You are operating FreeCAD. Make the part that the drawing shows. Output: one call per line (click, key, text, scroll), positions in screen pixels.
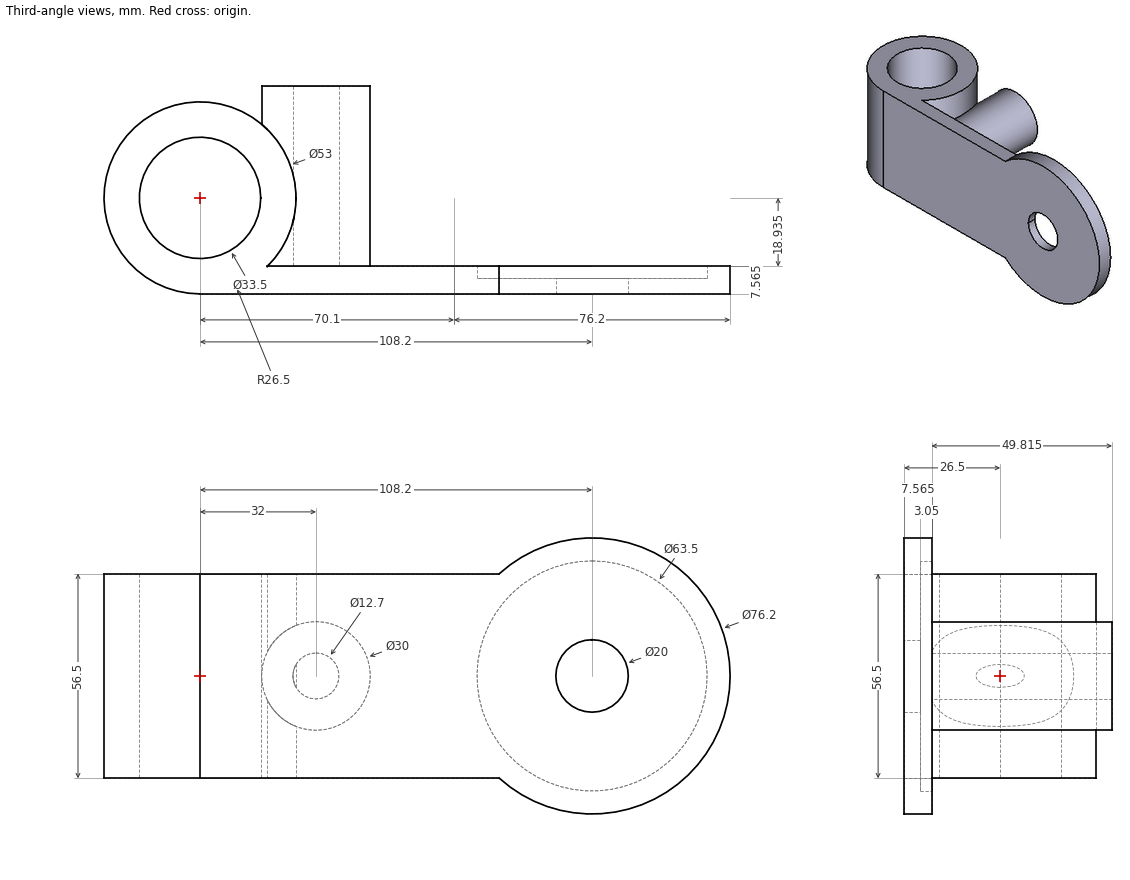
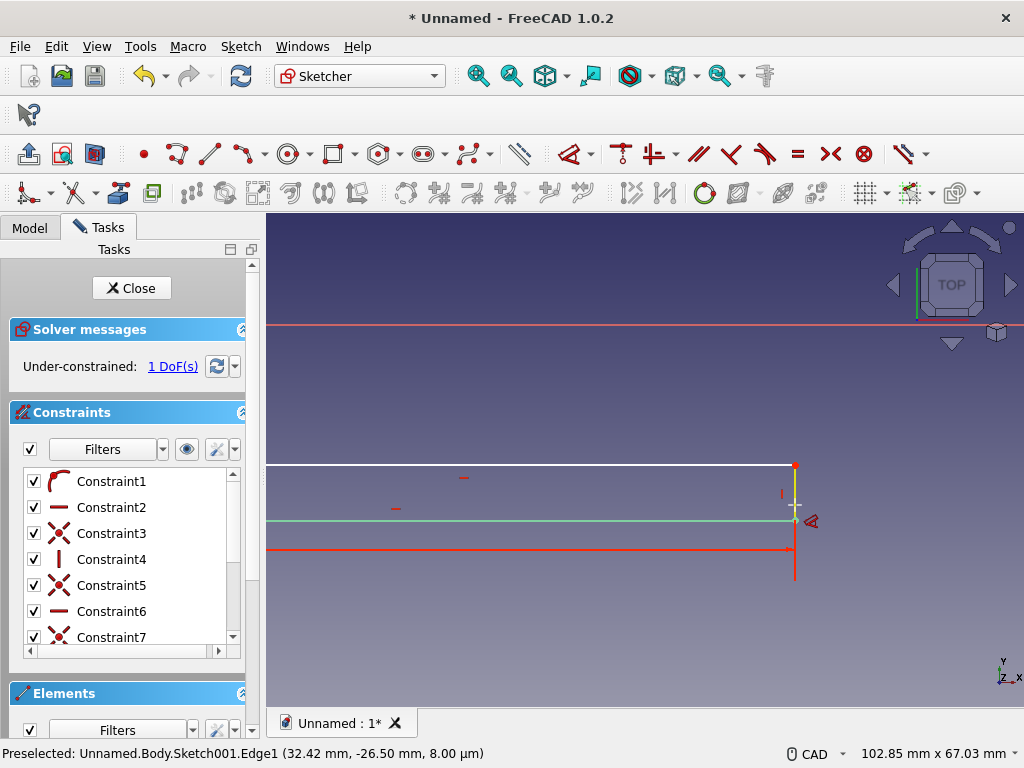
click(795, 504)
click(829, 493)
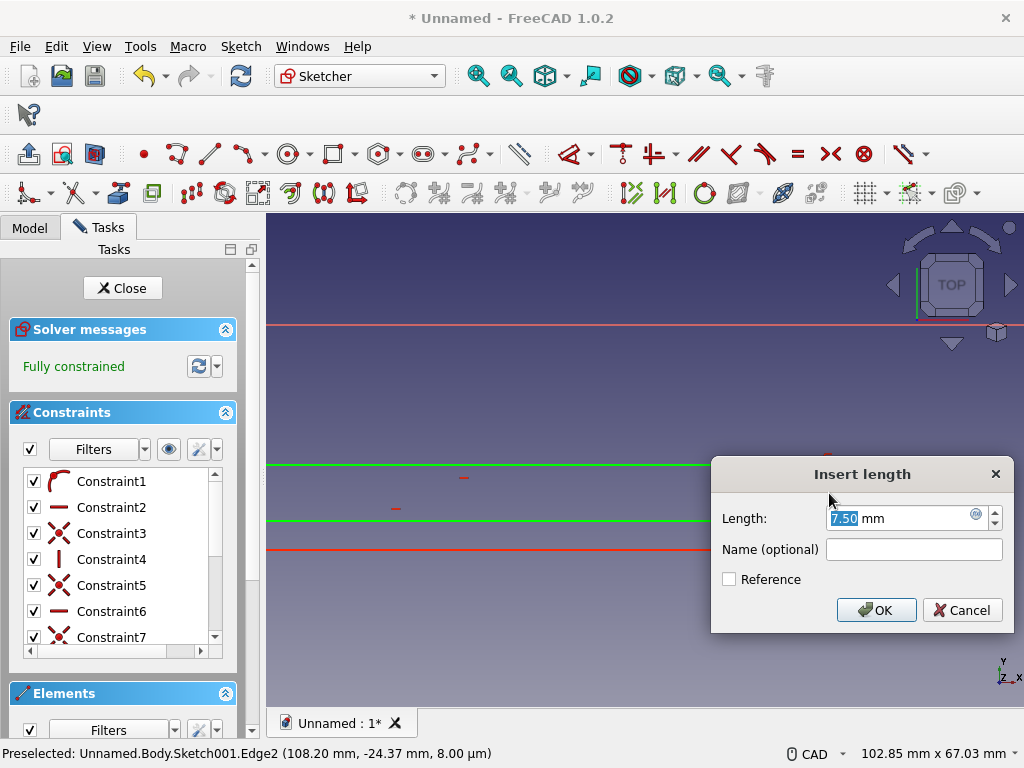
text(7.565)
key(Return)
key(Escape)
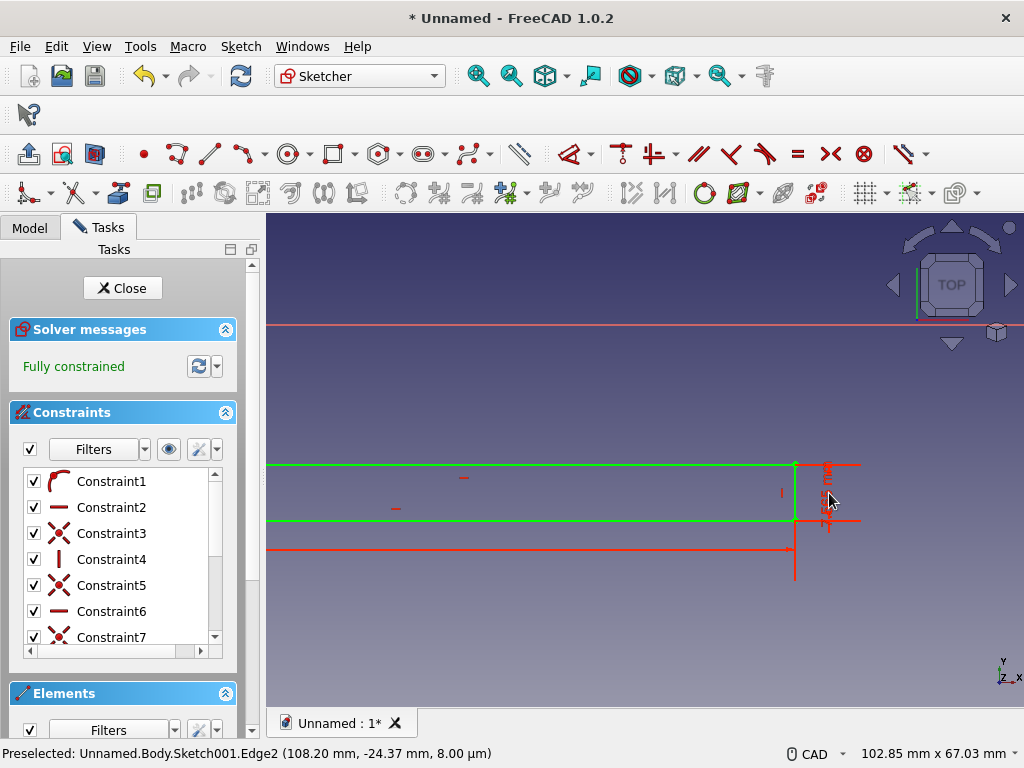
click(123, 288)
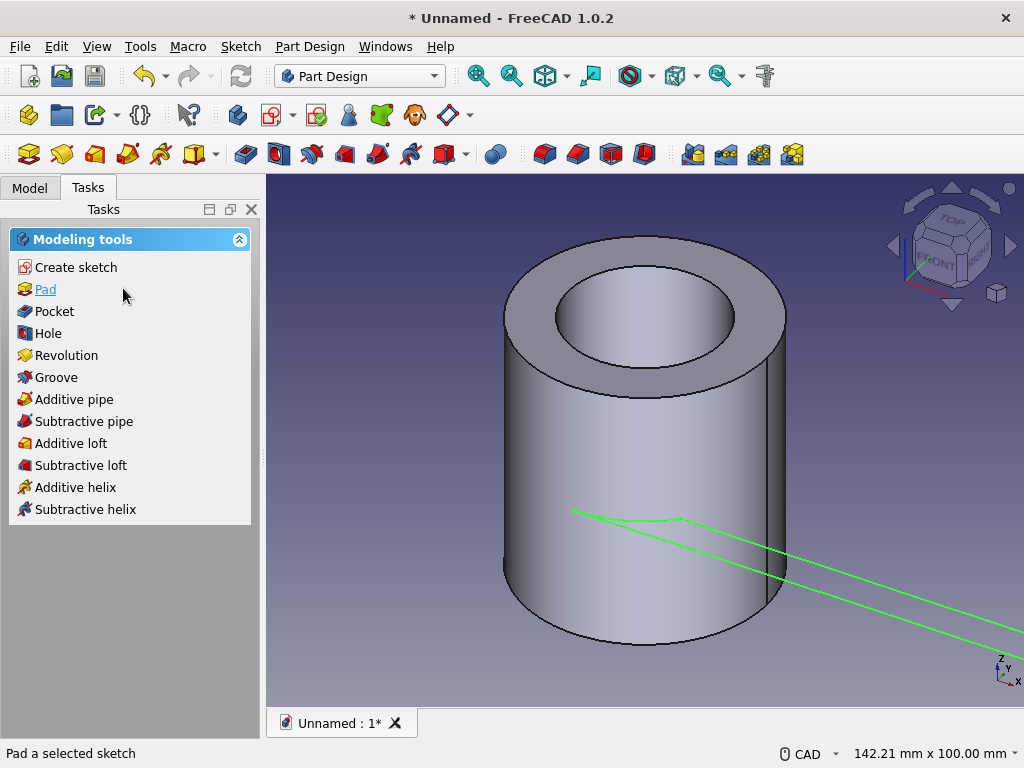
click(29, 154)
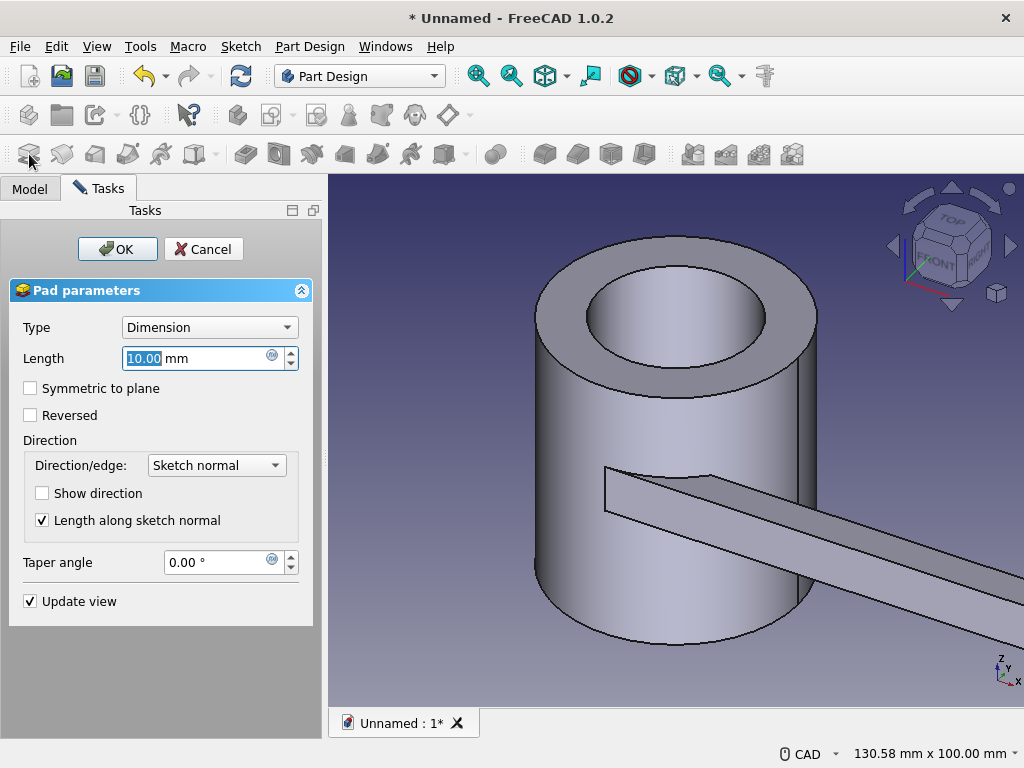
text(56.5)
key(Tab)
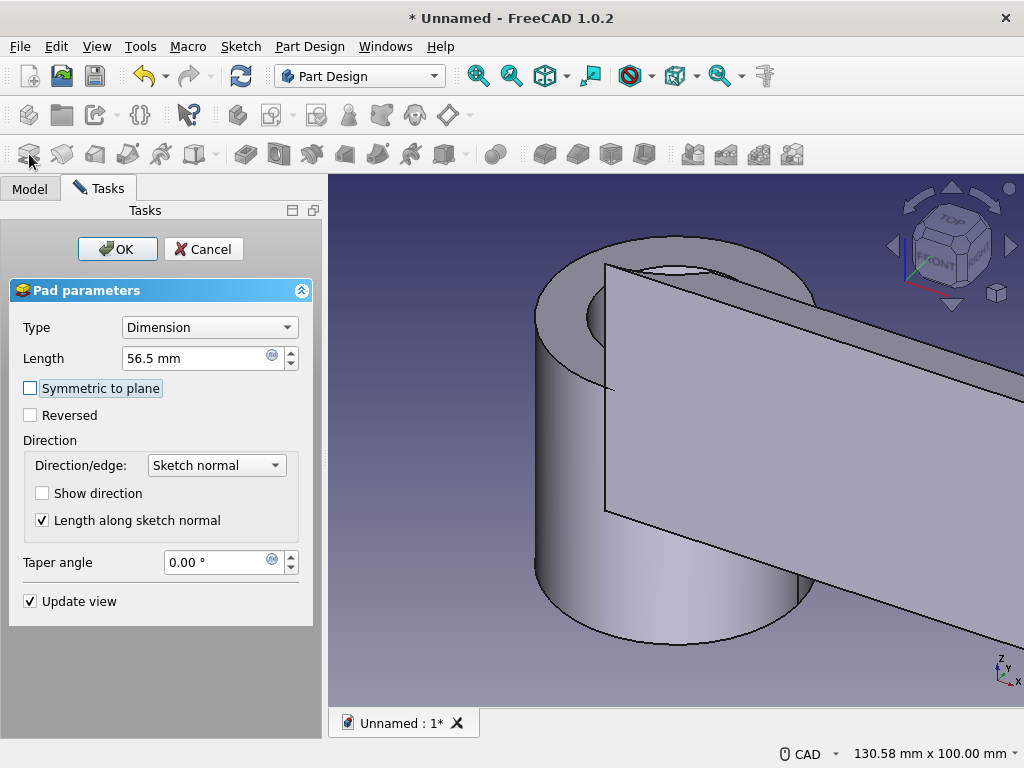
click(31, 388)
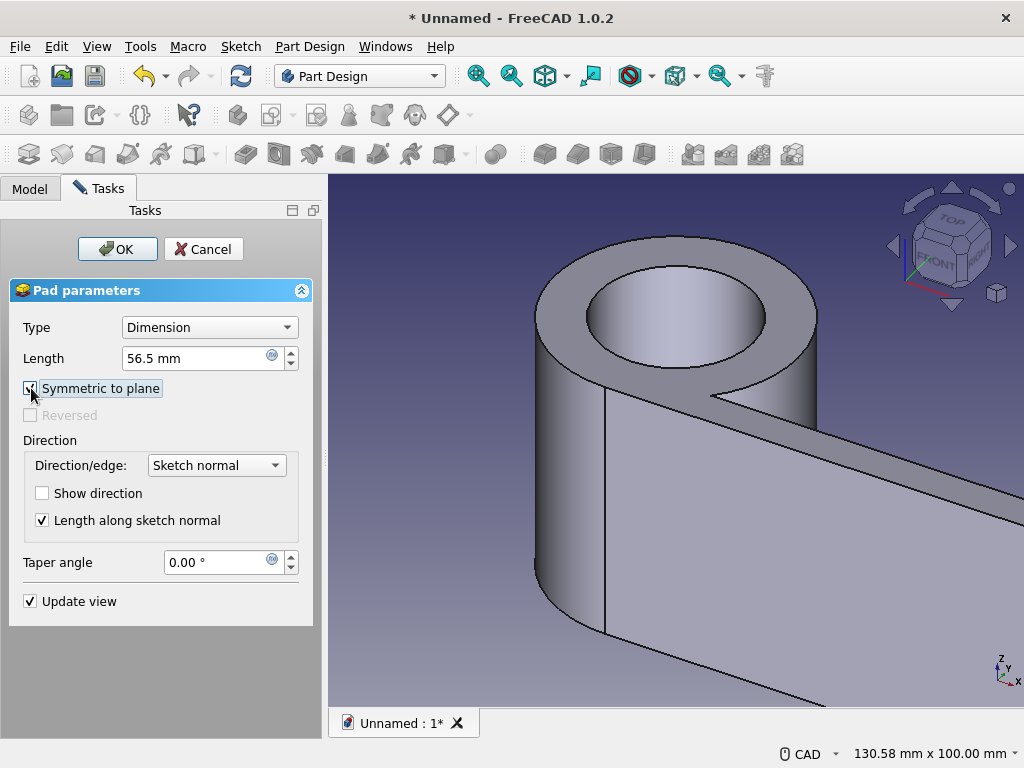
click(118, 249)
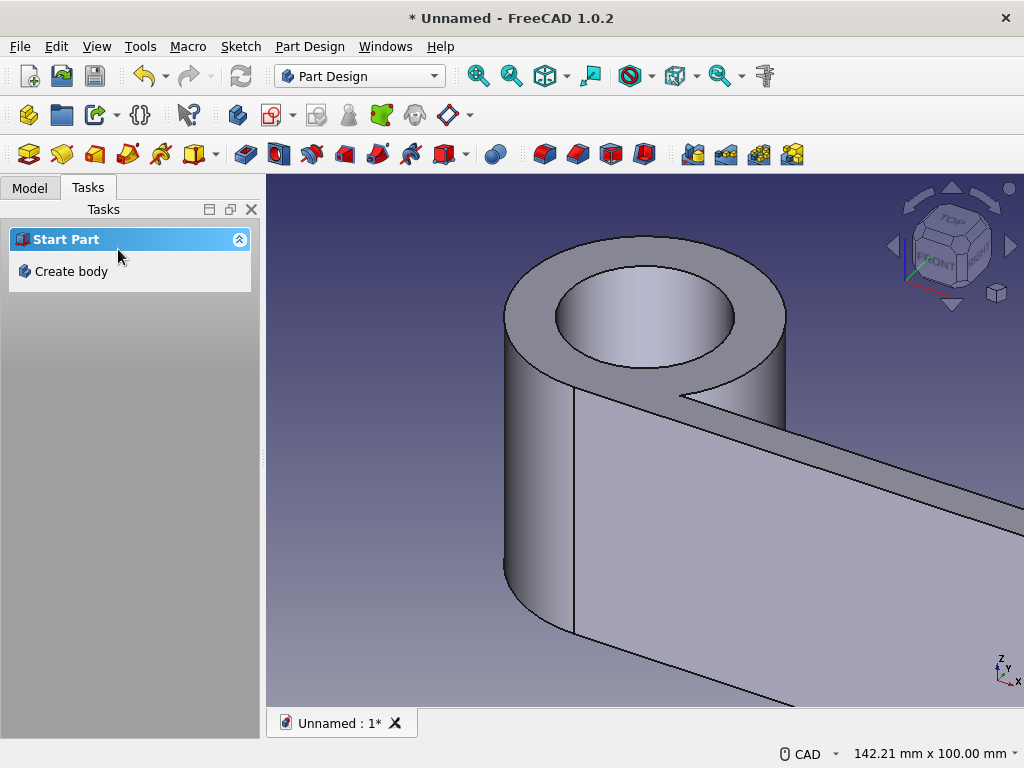
key(v)
key(f)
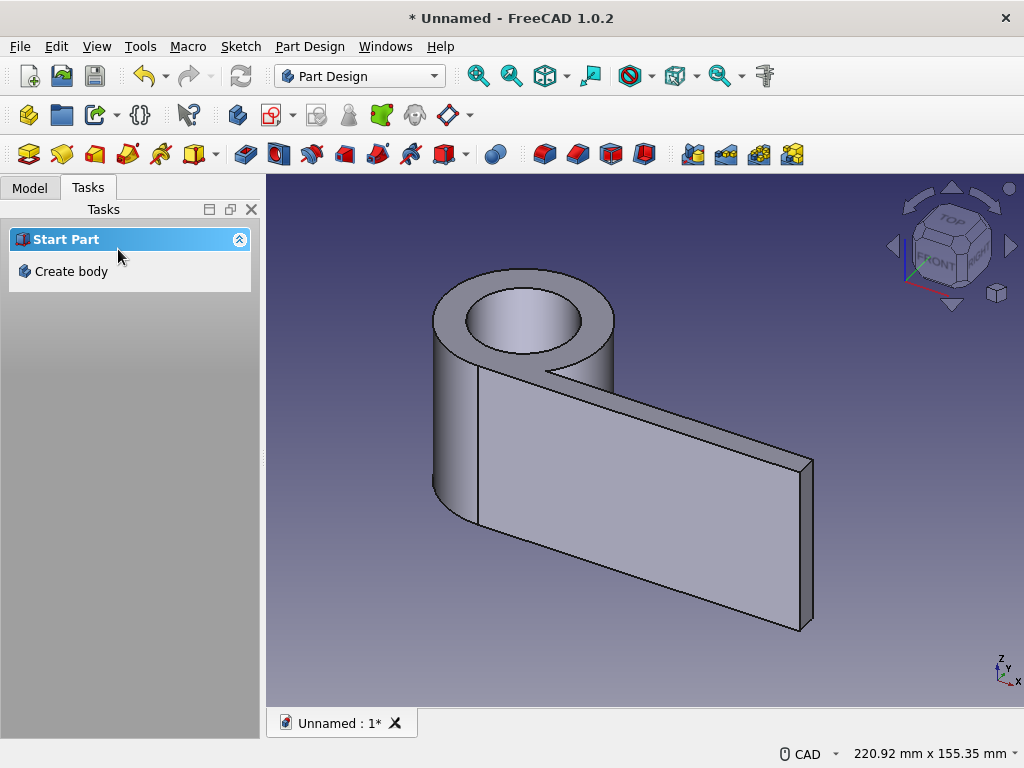
click(270, 116)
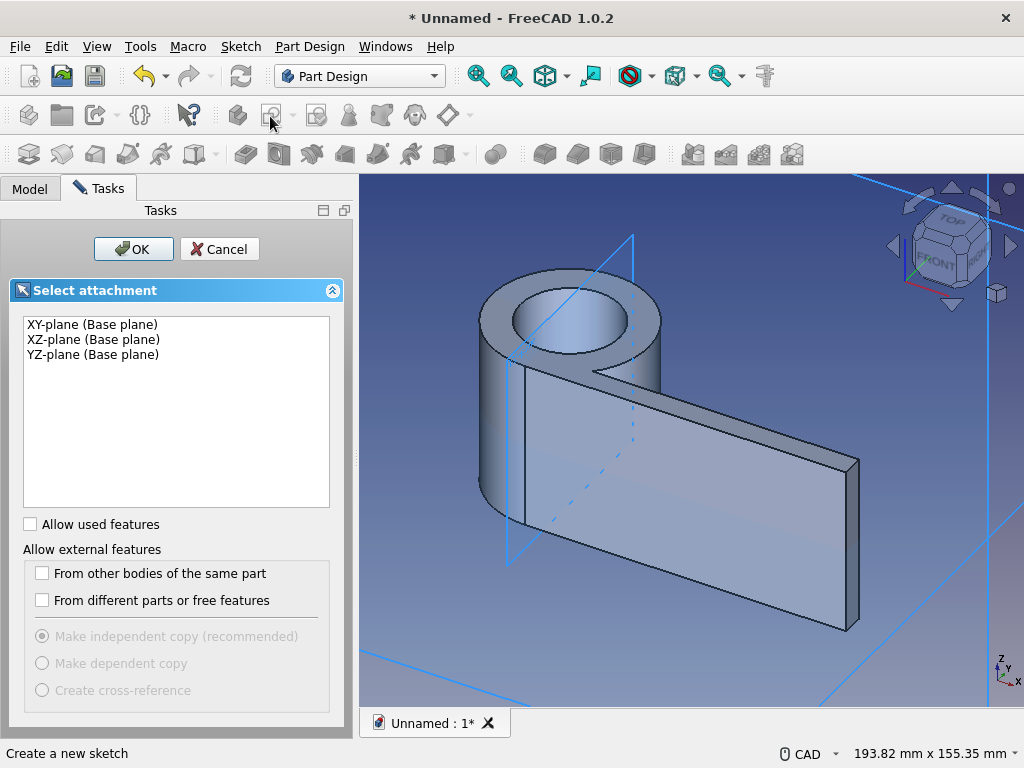
click(84, 340)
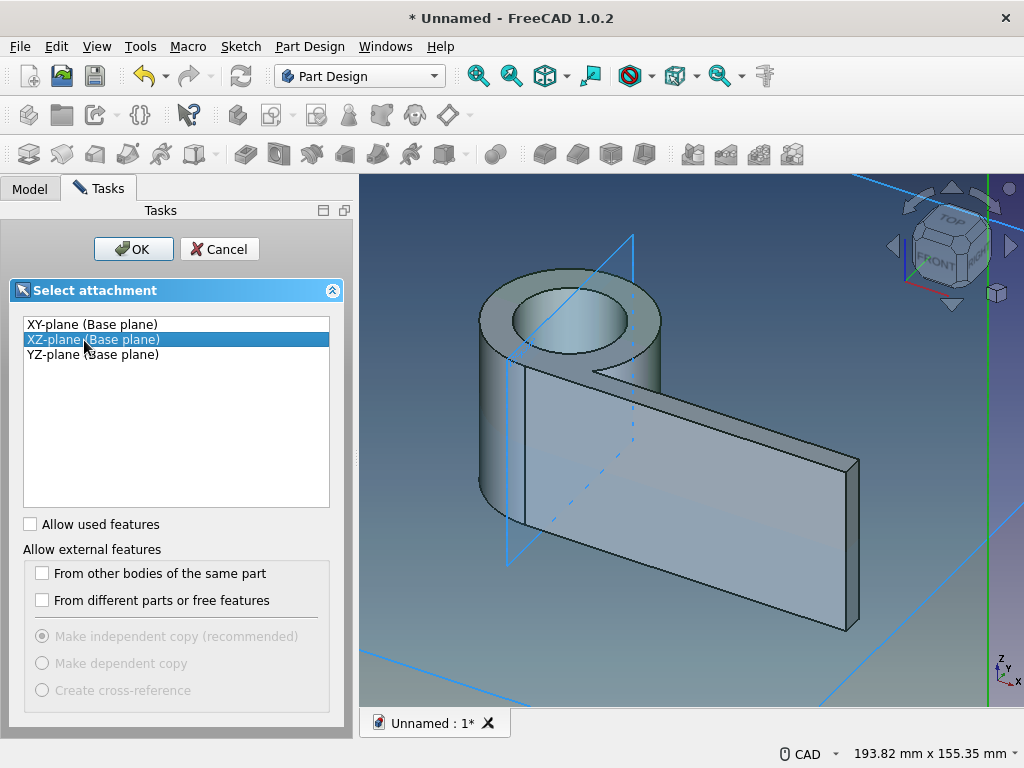
click(134, 249)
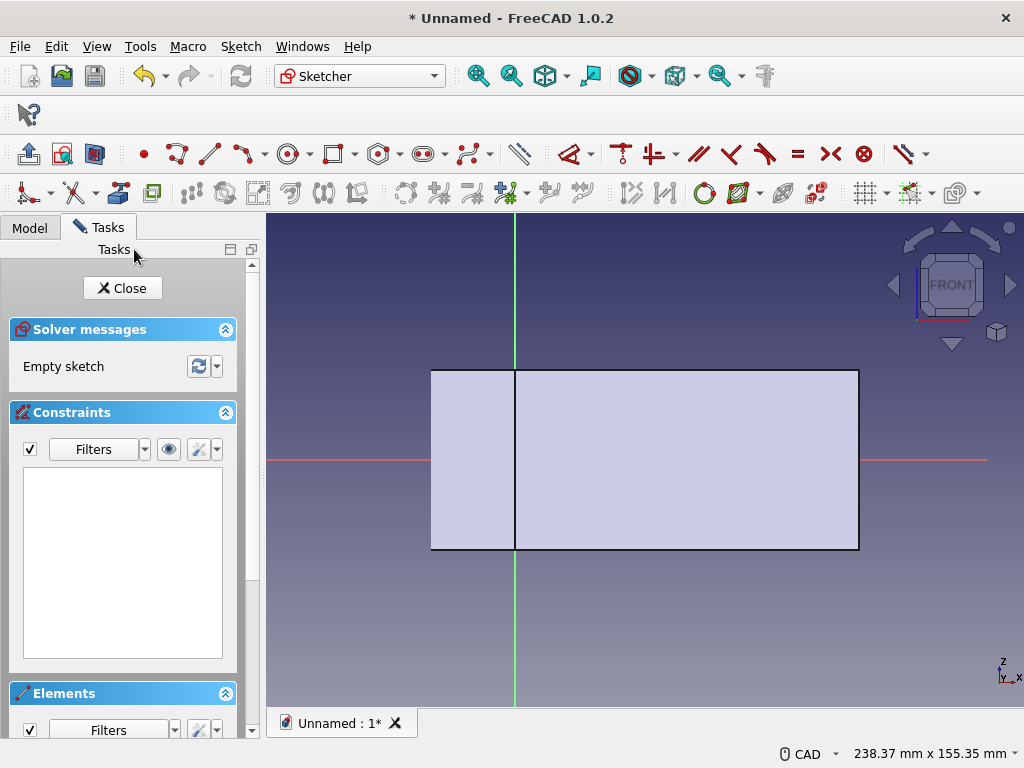
click(95, 154)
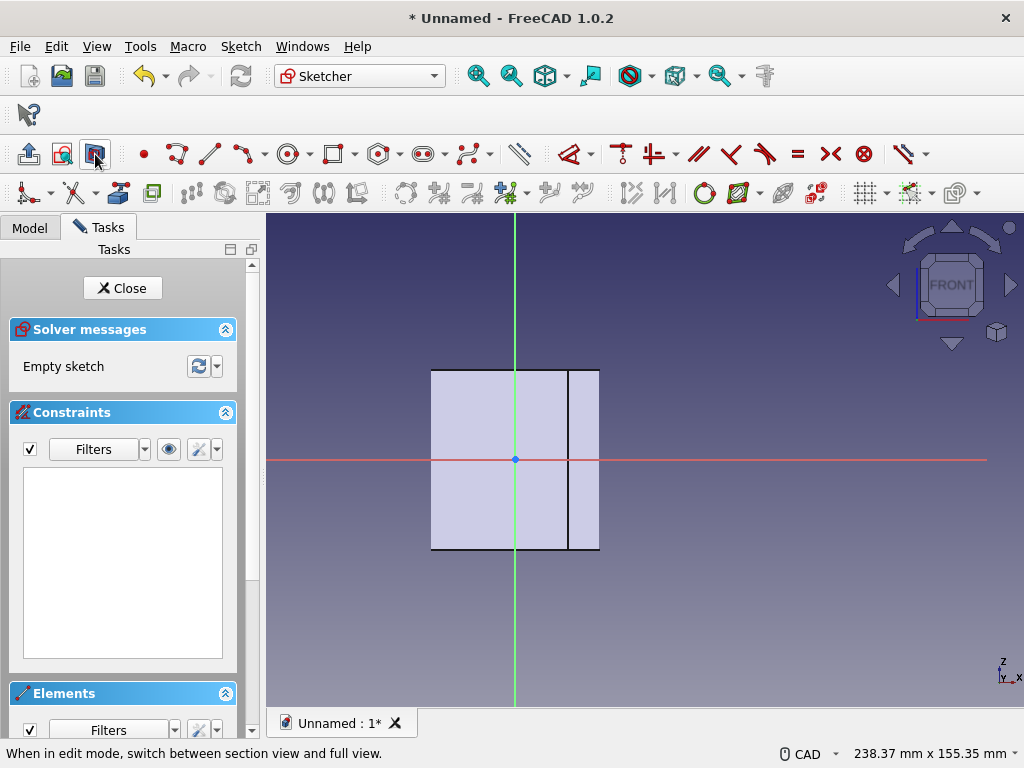
scroll(294, 460, down, 2)